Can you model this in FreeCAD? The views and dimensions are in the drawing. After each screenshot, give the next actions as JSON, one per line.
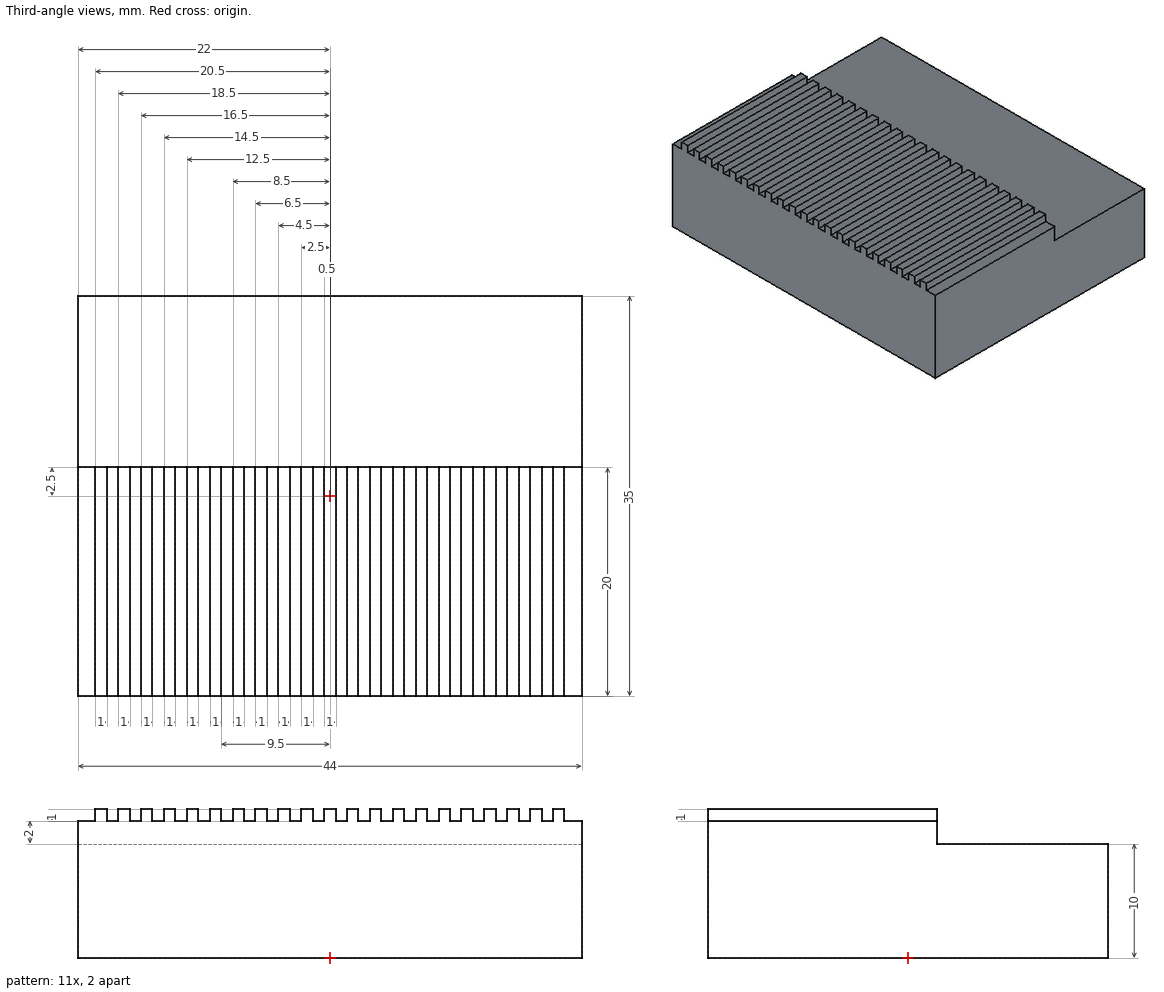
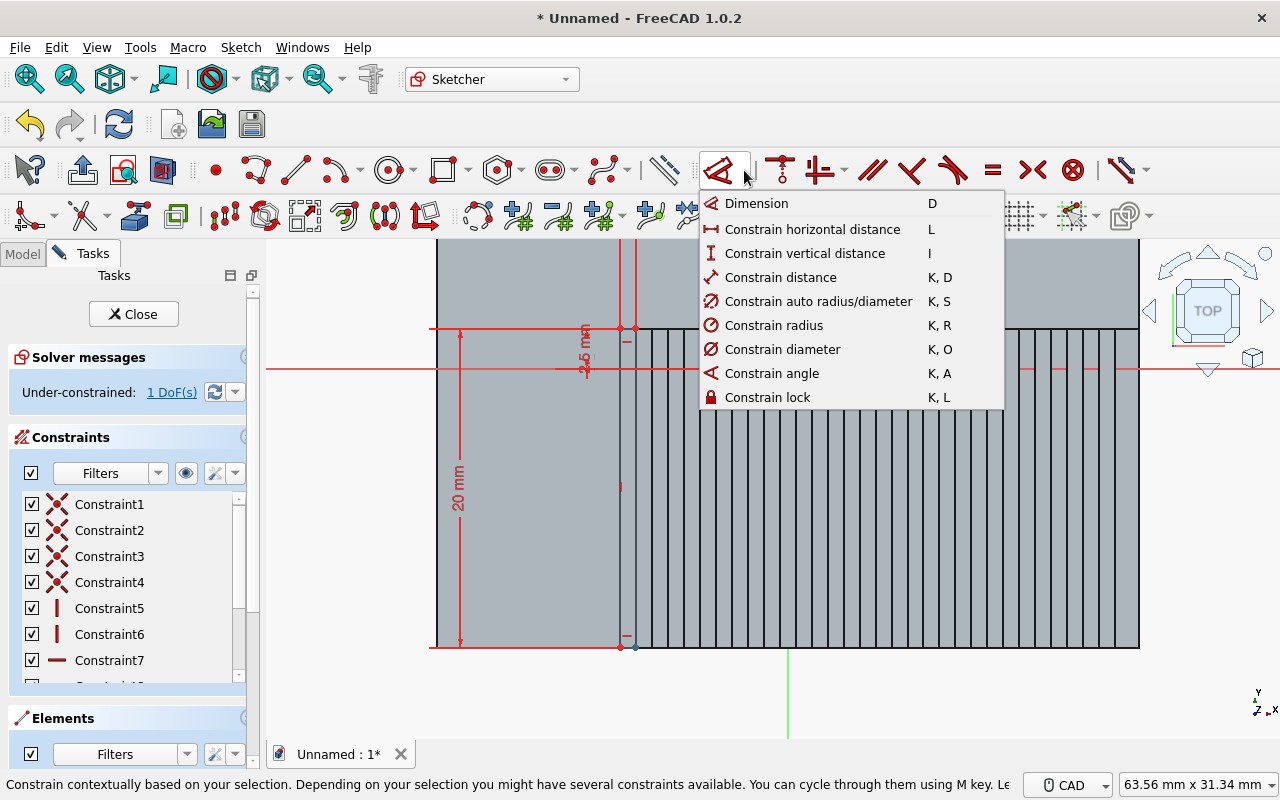
{"action": "left_click", "coordinate": [852, 229]}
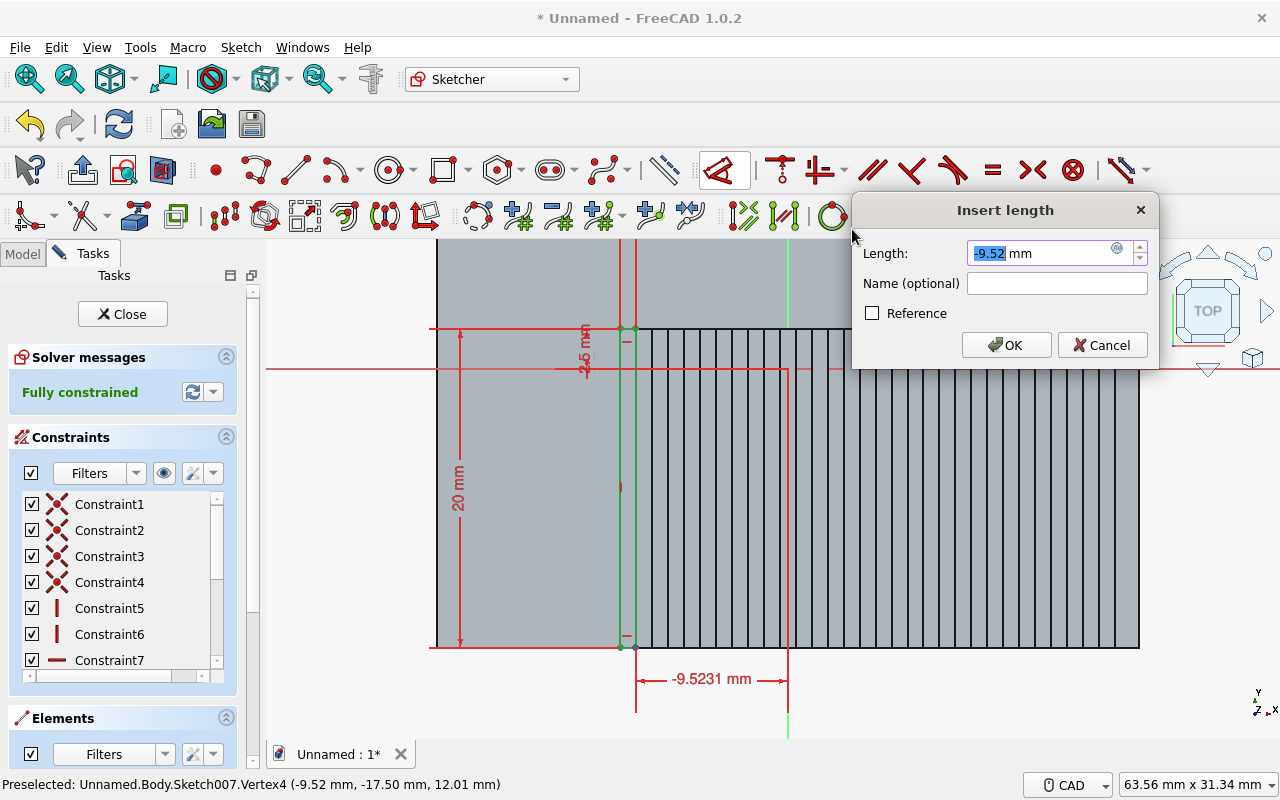
{"action": "type", "text": "-9.5"}
{"action": "key", "text": "Return"}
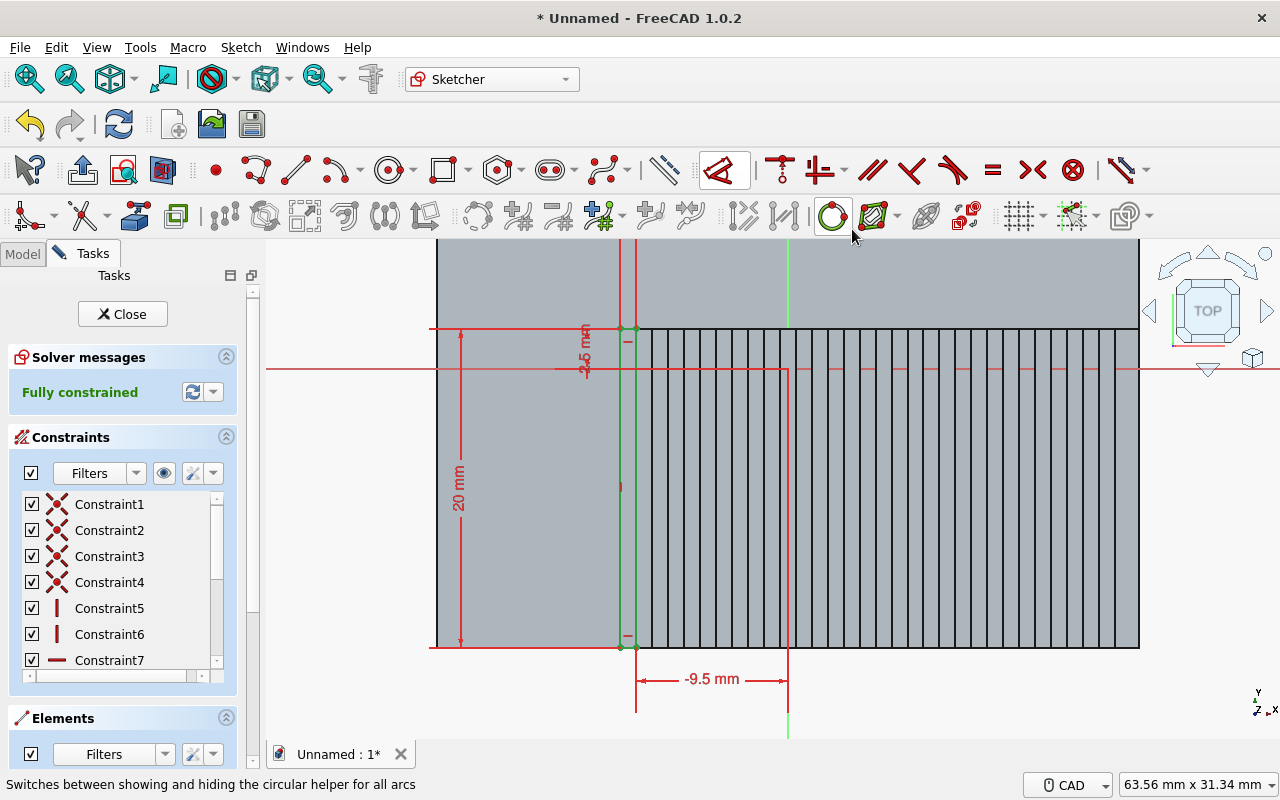
{"action": "left_click", "coordinate": [123, 314]}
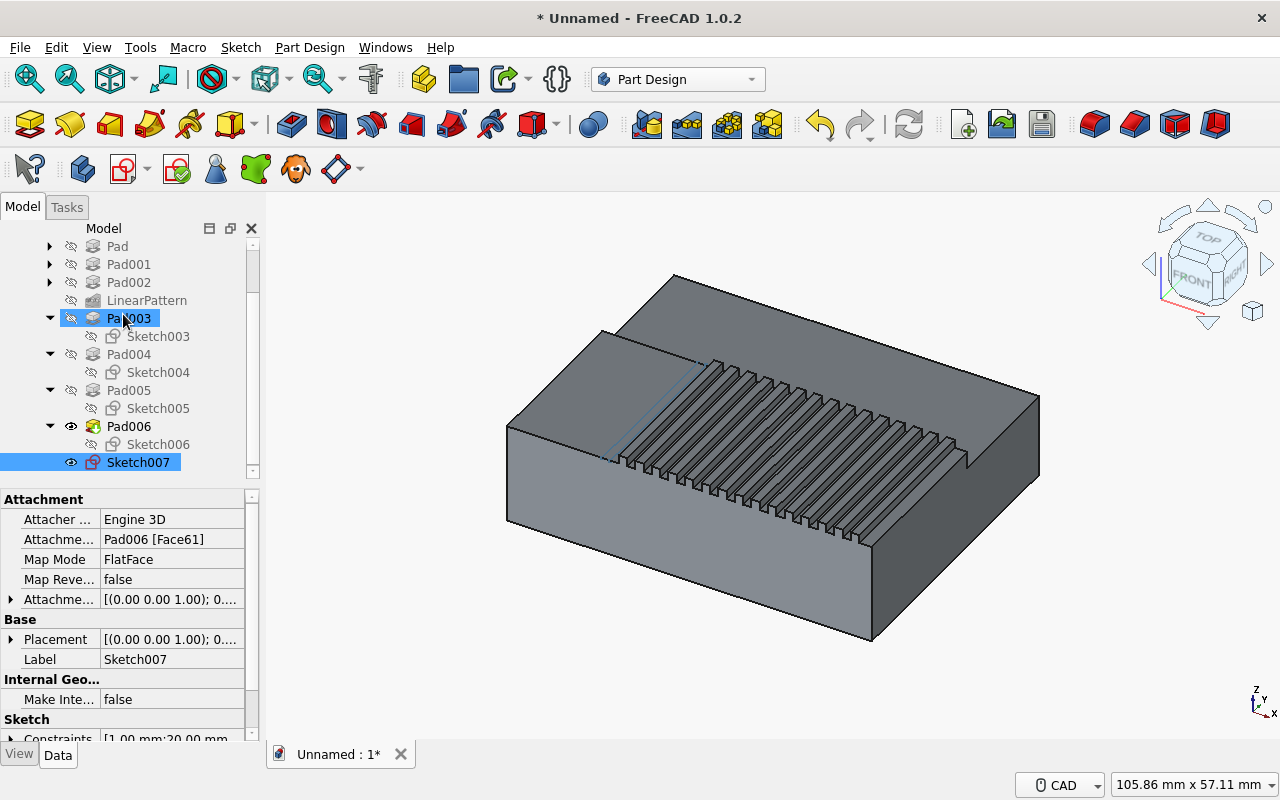
{"action": "left_click", "coordinate": [30, 124]}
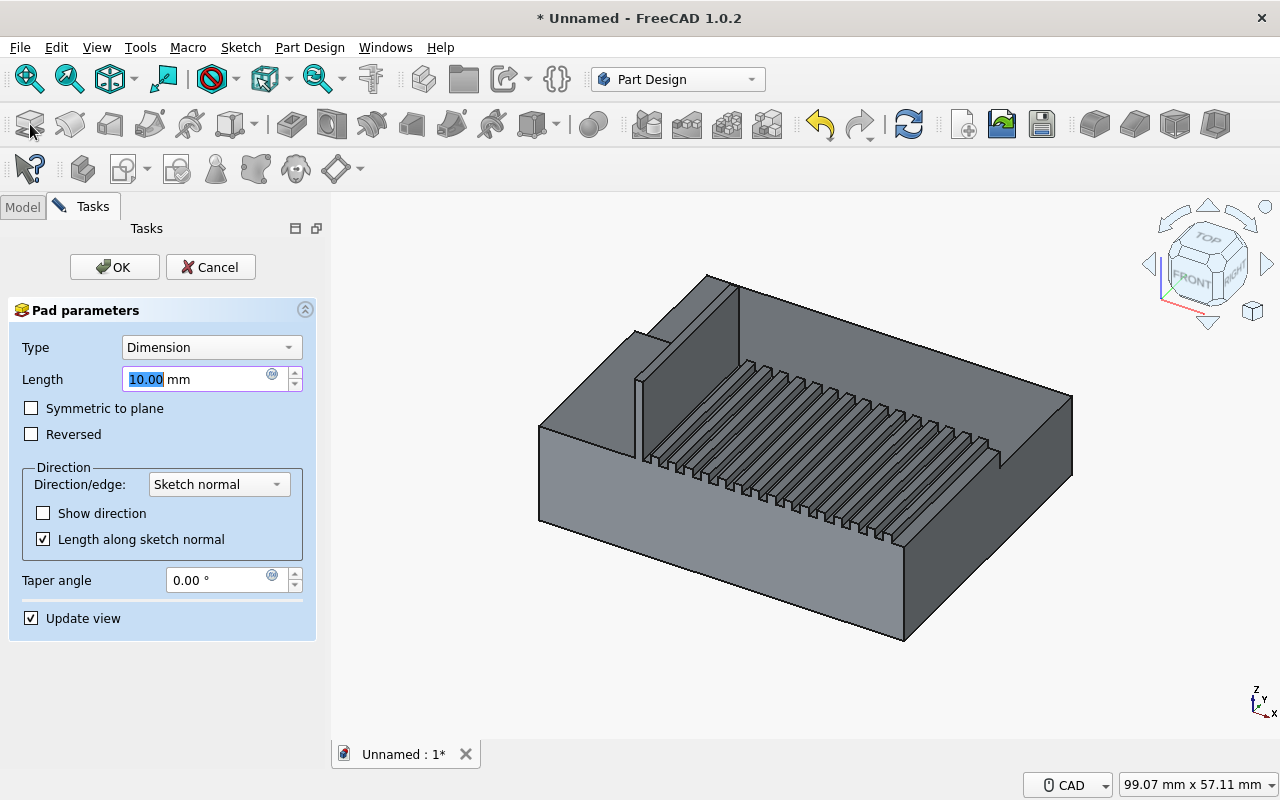
{"action": "type", "text": "1"}
{"action": "key", "text": "Tab"}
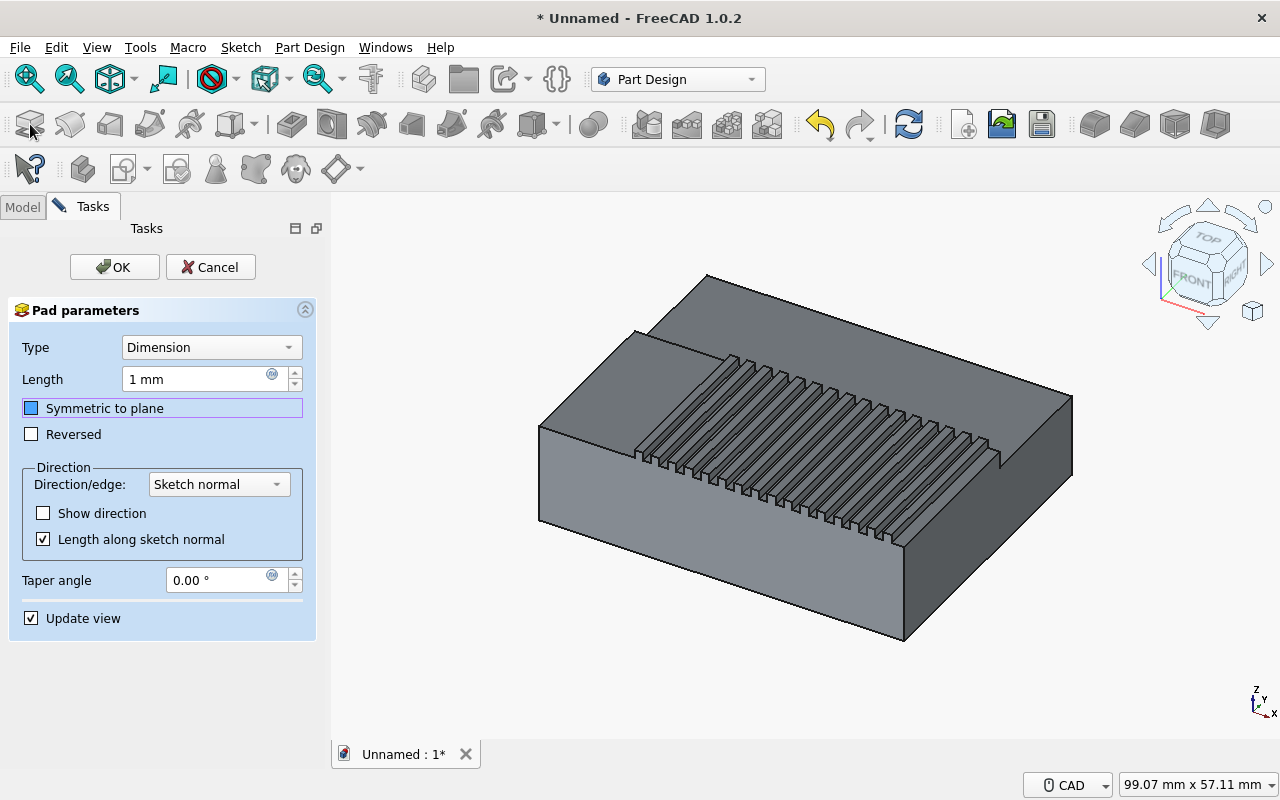
{"action": "left_click", "coordinate": [115, 267]}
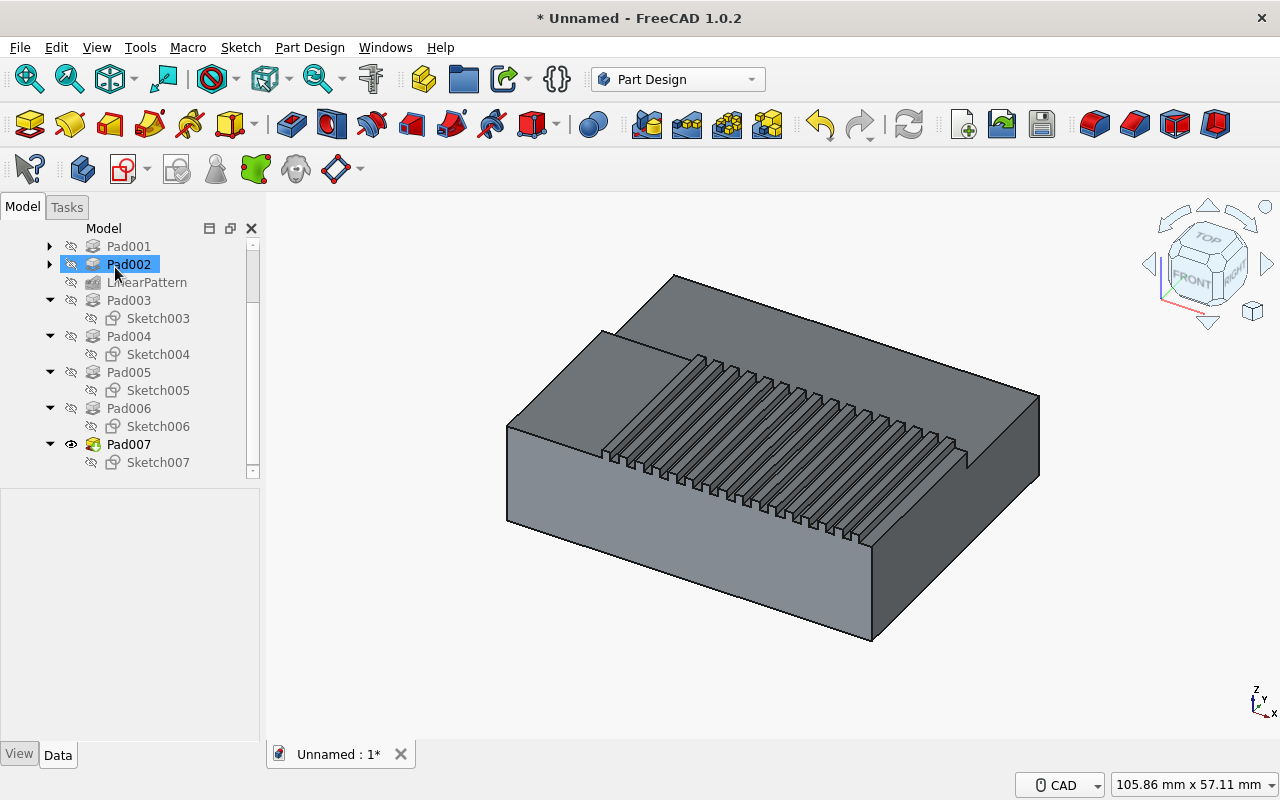
{"action": "left_click", "coordinate": [616, 380]}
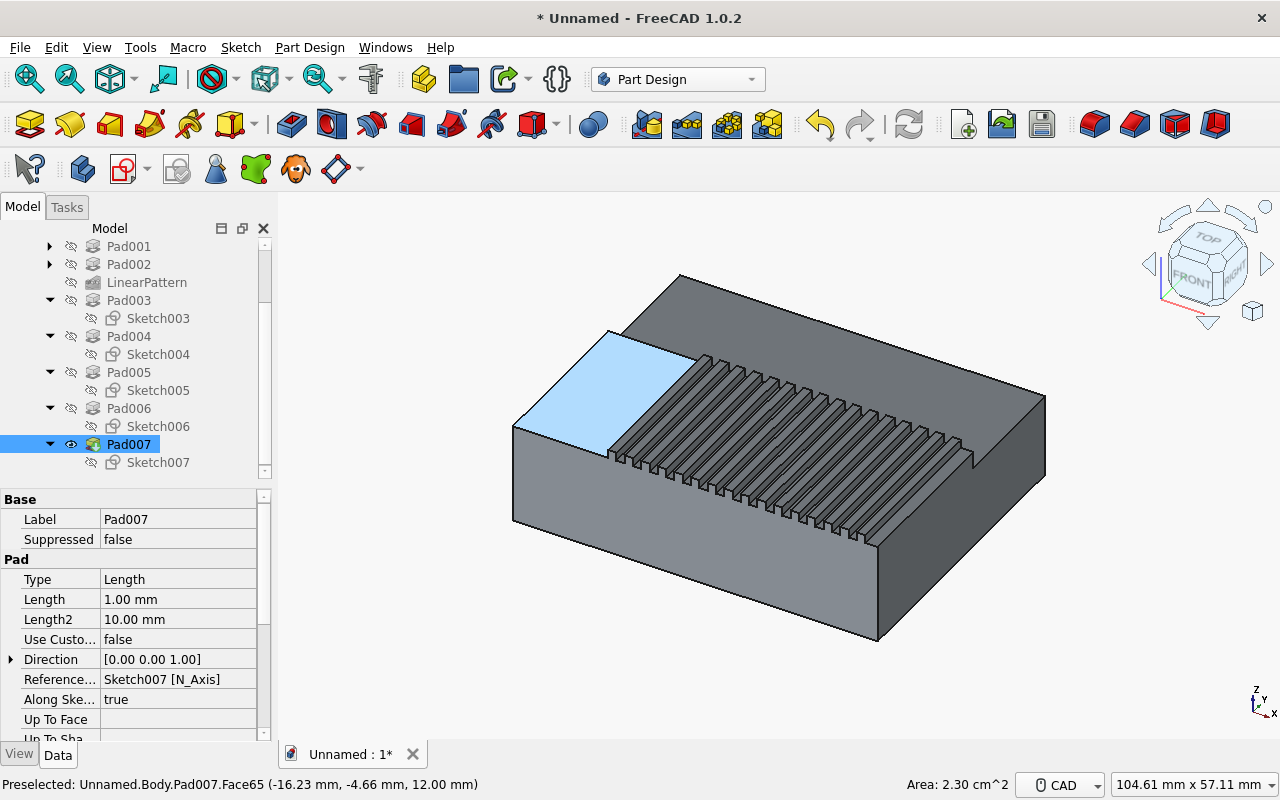
{"action": "left_click", "coordinate": [124, 170]}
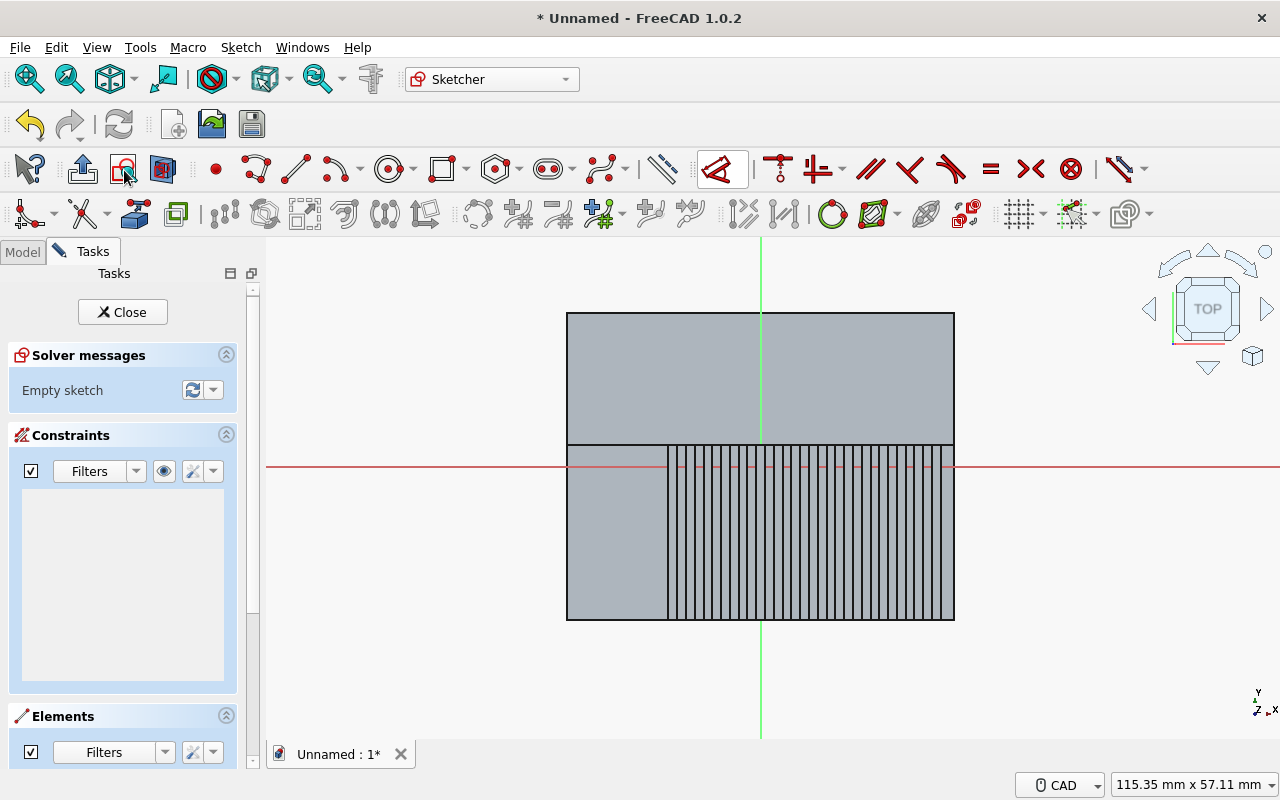
{"action": "left_click", "coordinate": [164, 170]}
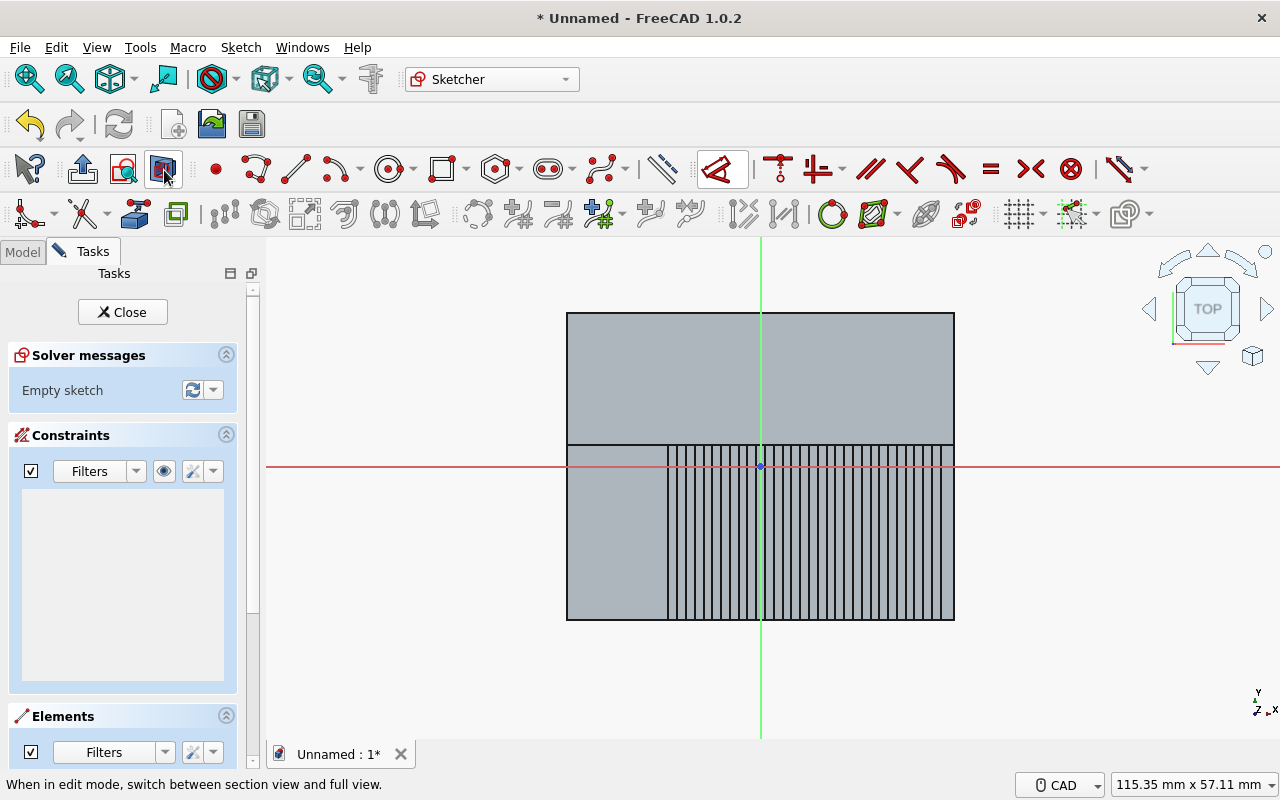
{"action": "scroll", "coordinate": [707, 587], "scroll_direction": "up", "scroll_amount": 3}